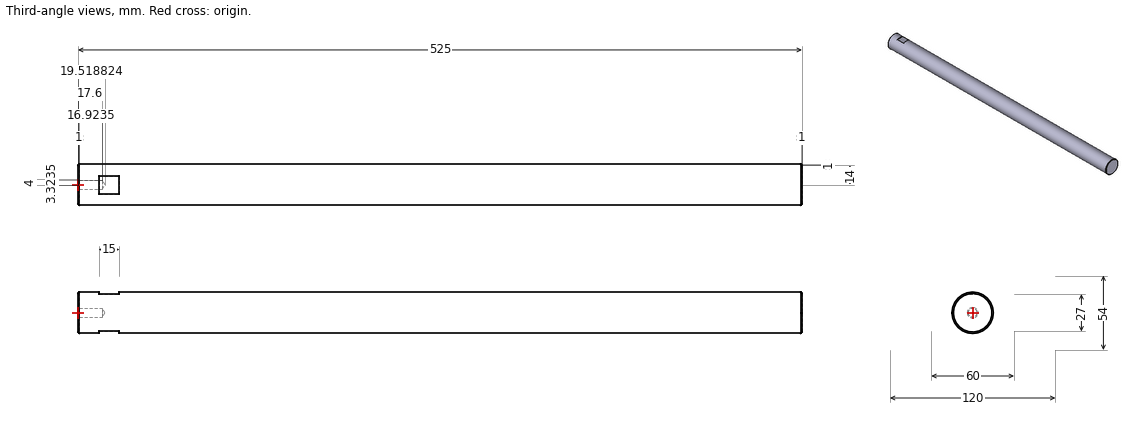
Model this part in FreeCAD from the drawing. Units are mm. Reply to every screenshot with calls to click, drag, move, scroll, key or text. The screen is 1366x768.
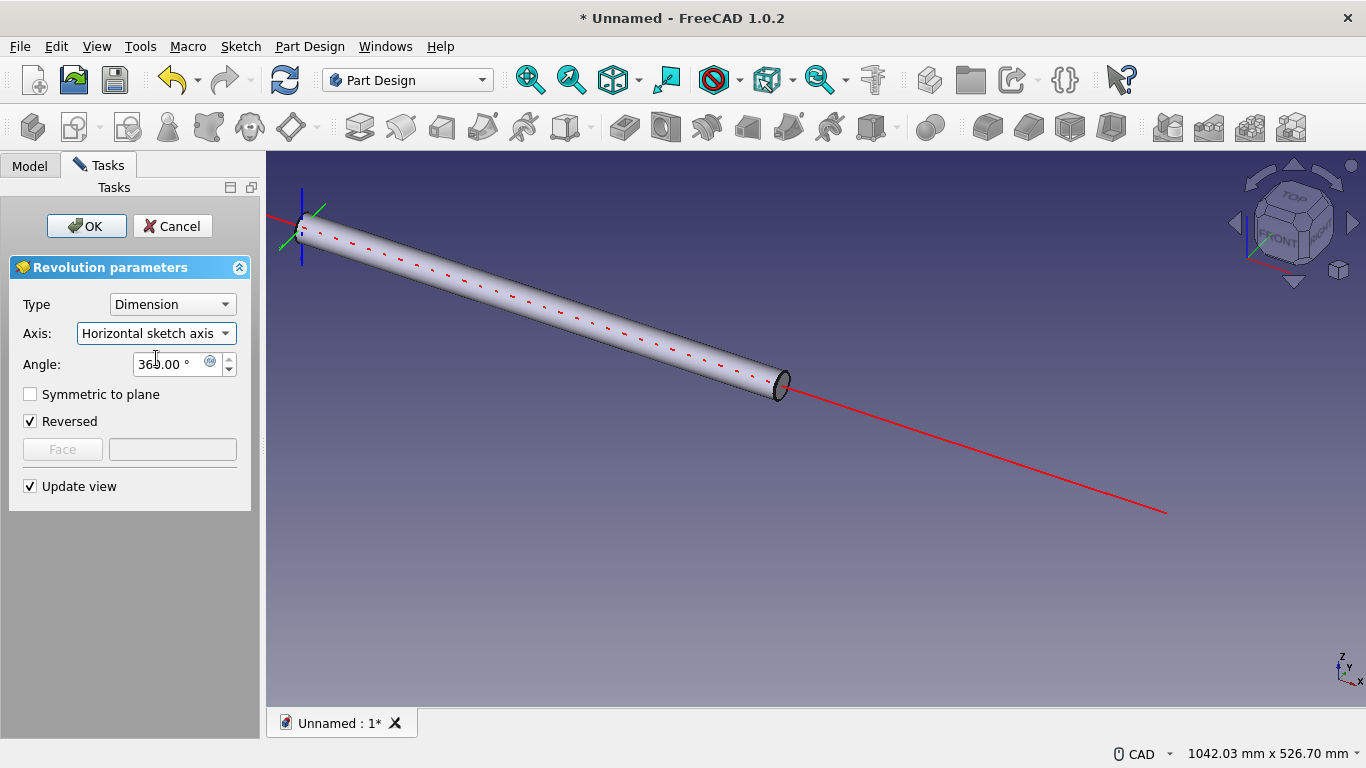
click(87, 226)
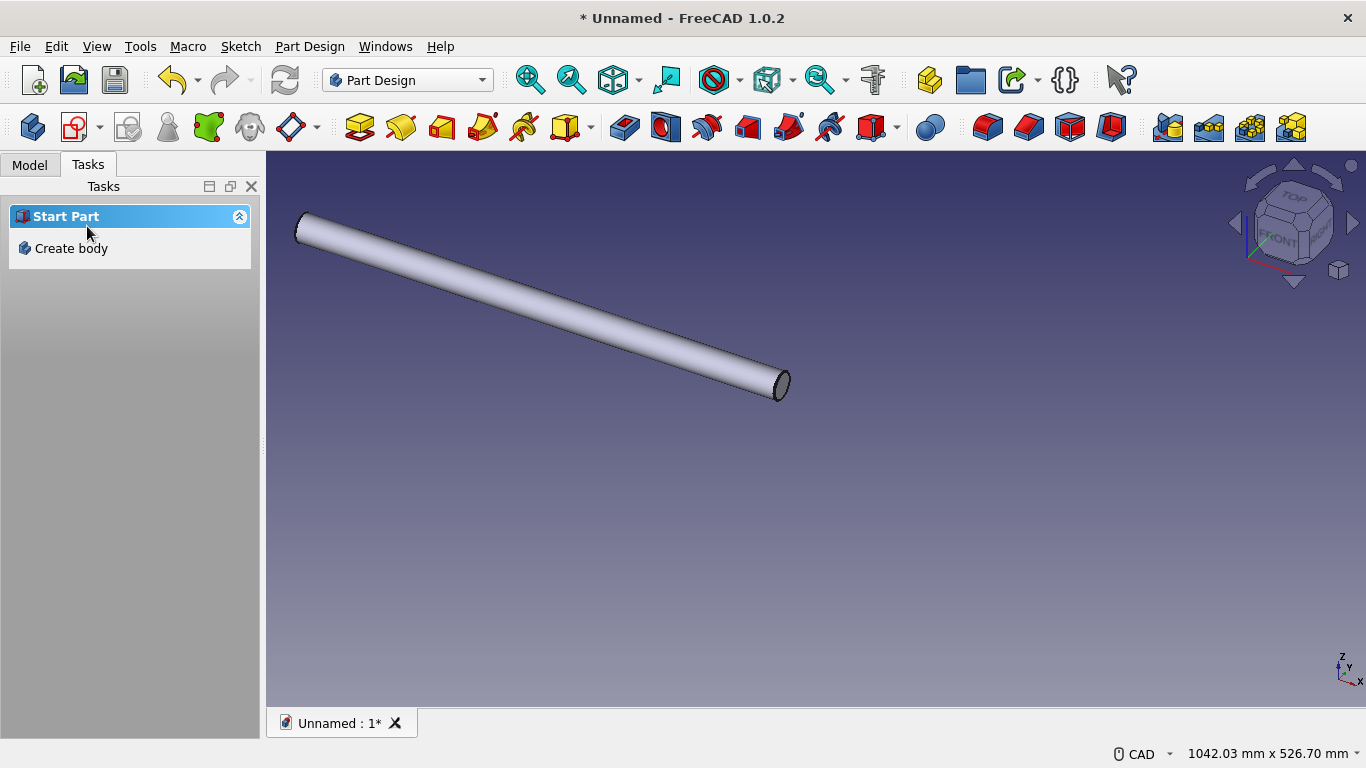
click(30, 164)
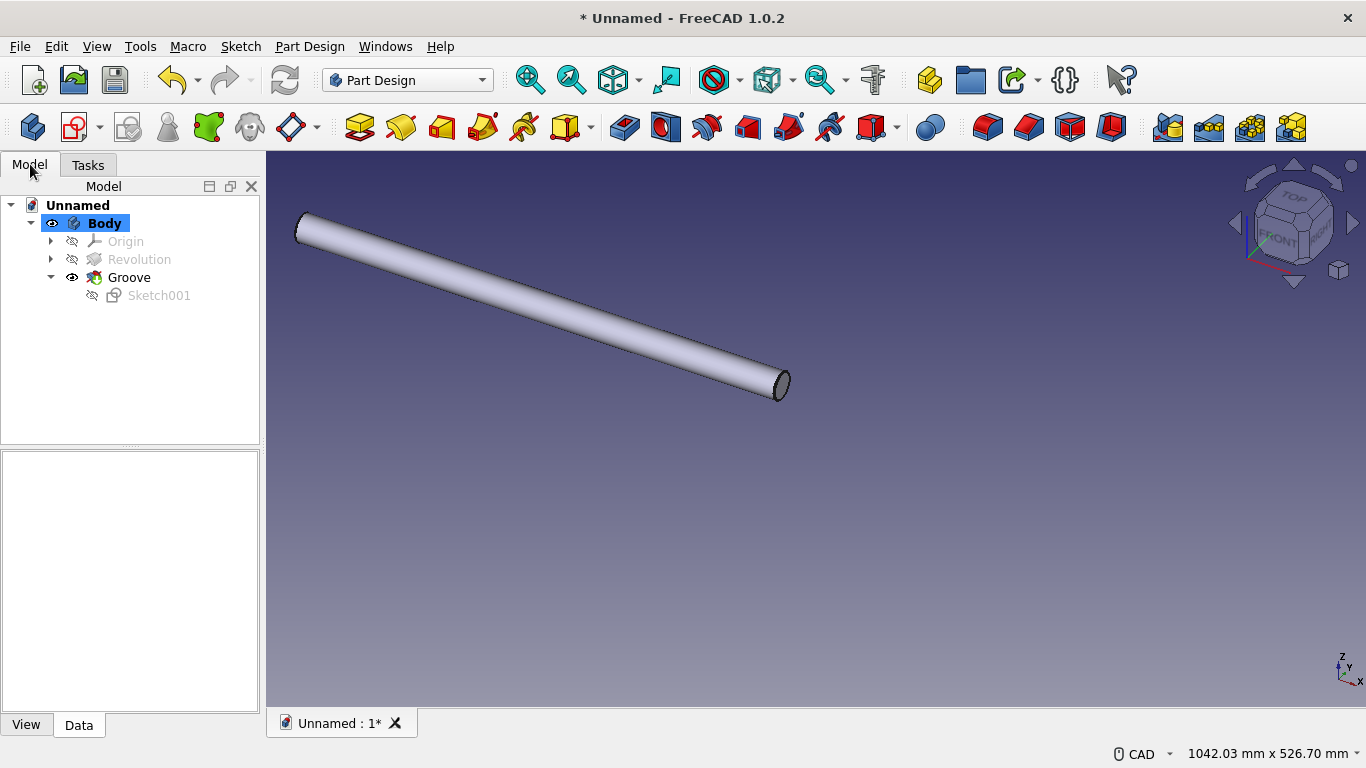
click(51, 241)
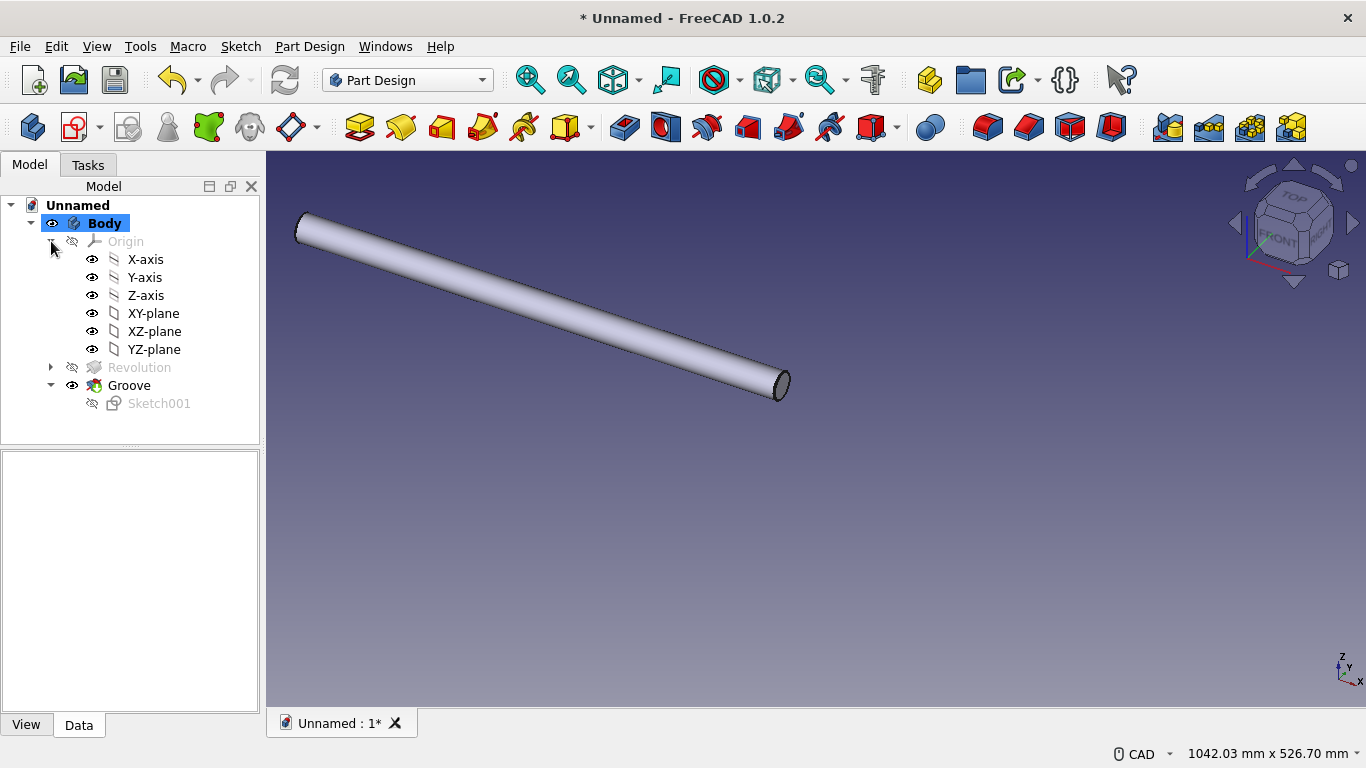
click(137, 349)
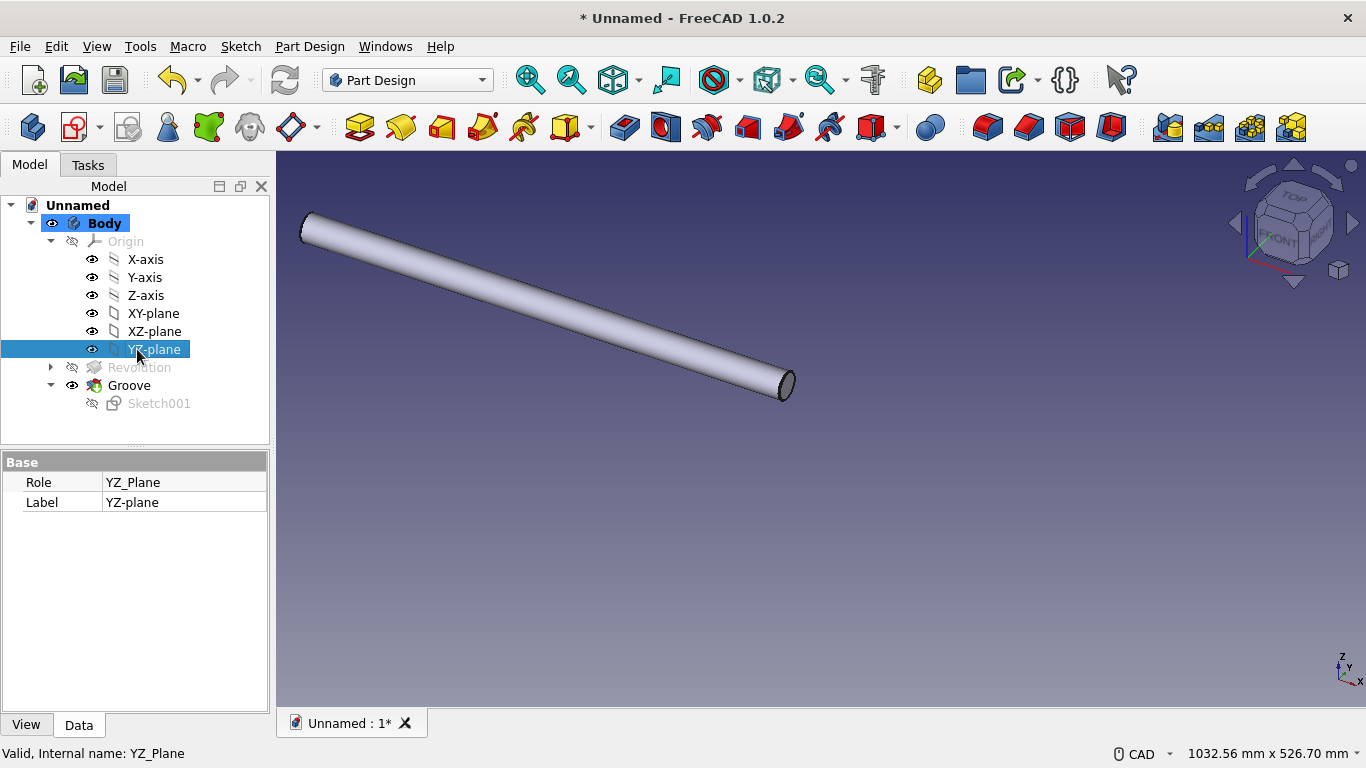
click(290, 128)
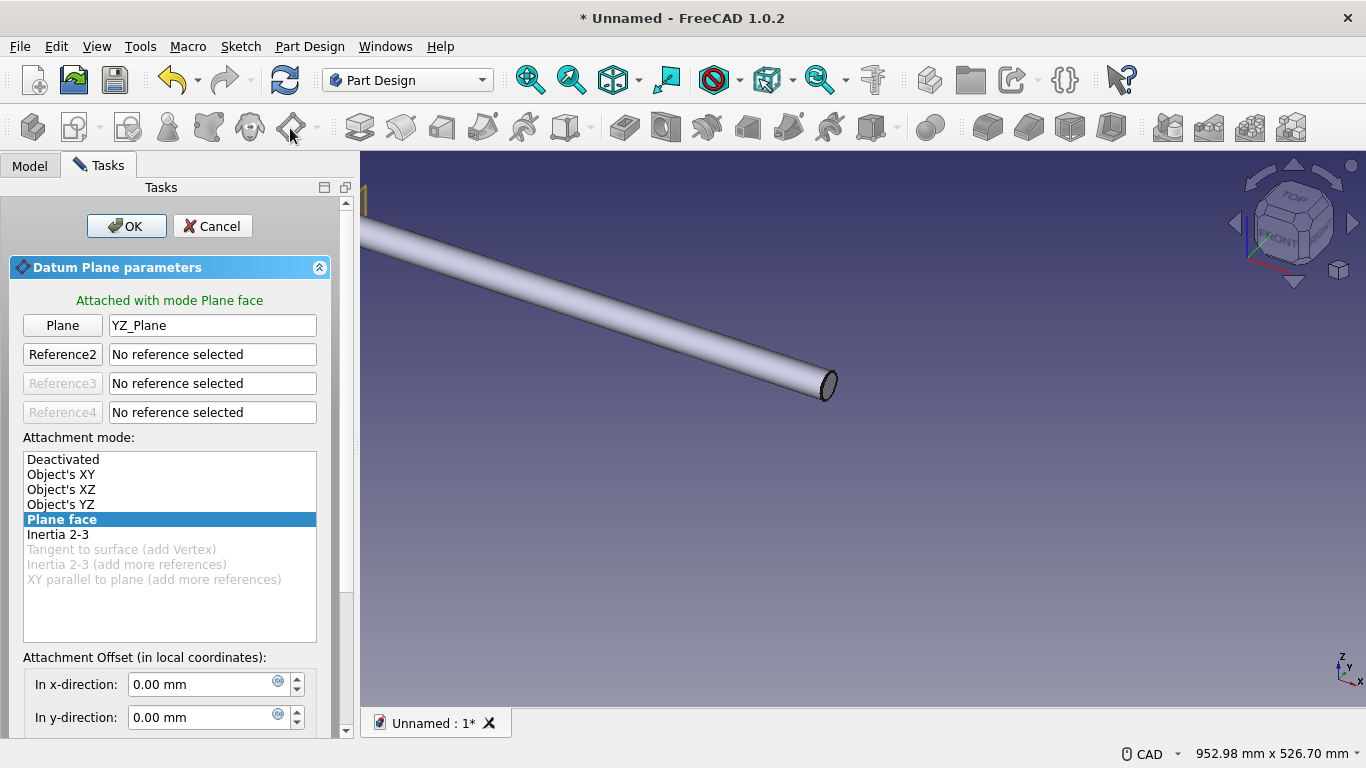
scroll(346, 468, down, 2)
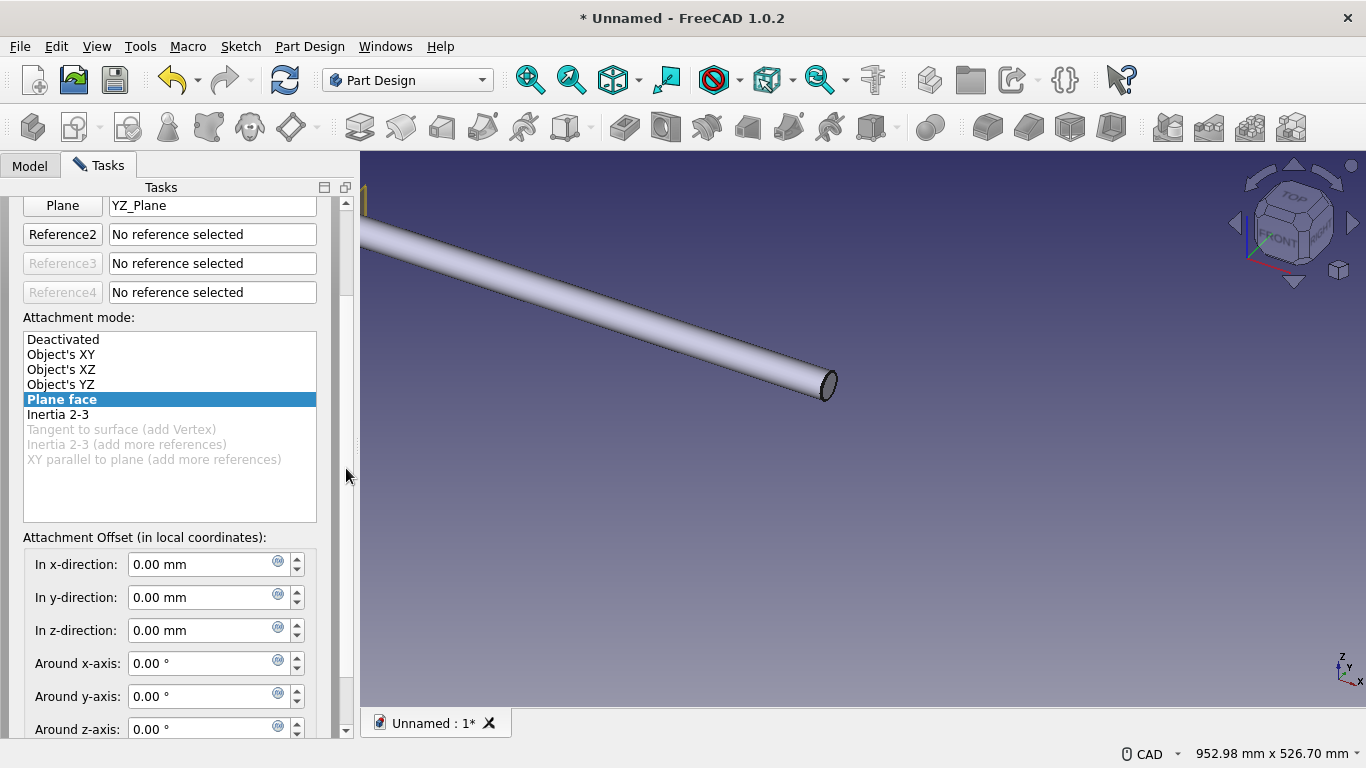
triple_click(210, 630)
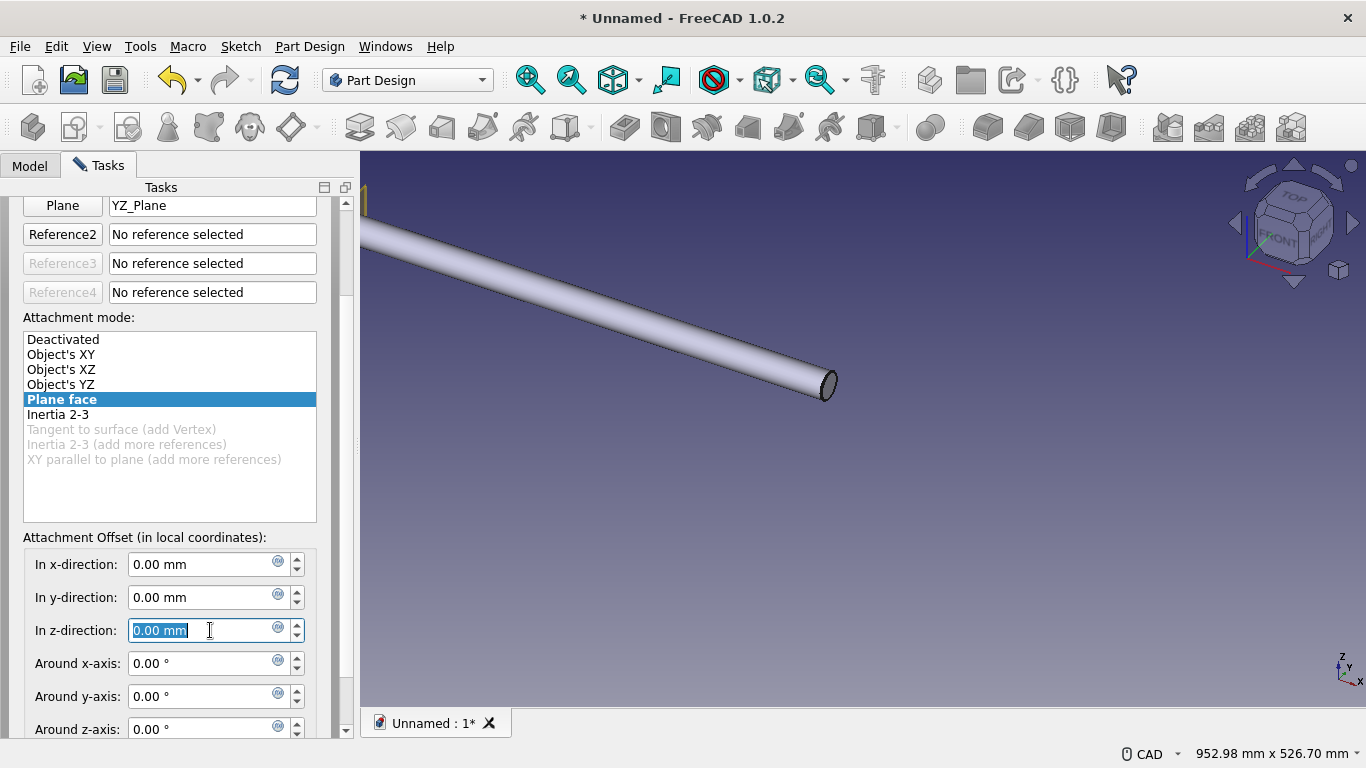
text(15)
key(Tab)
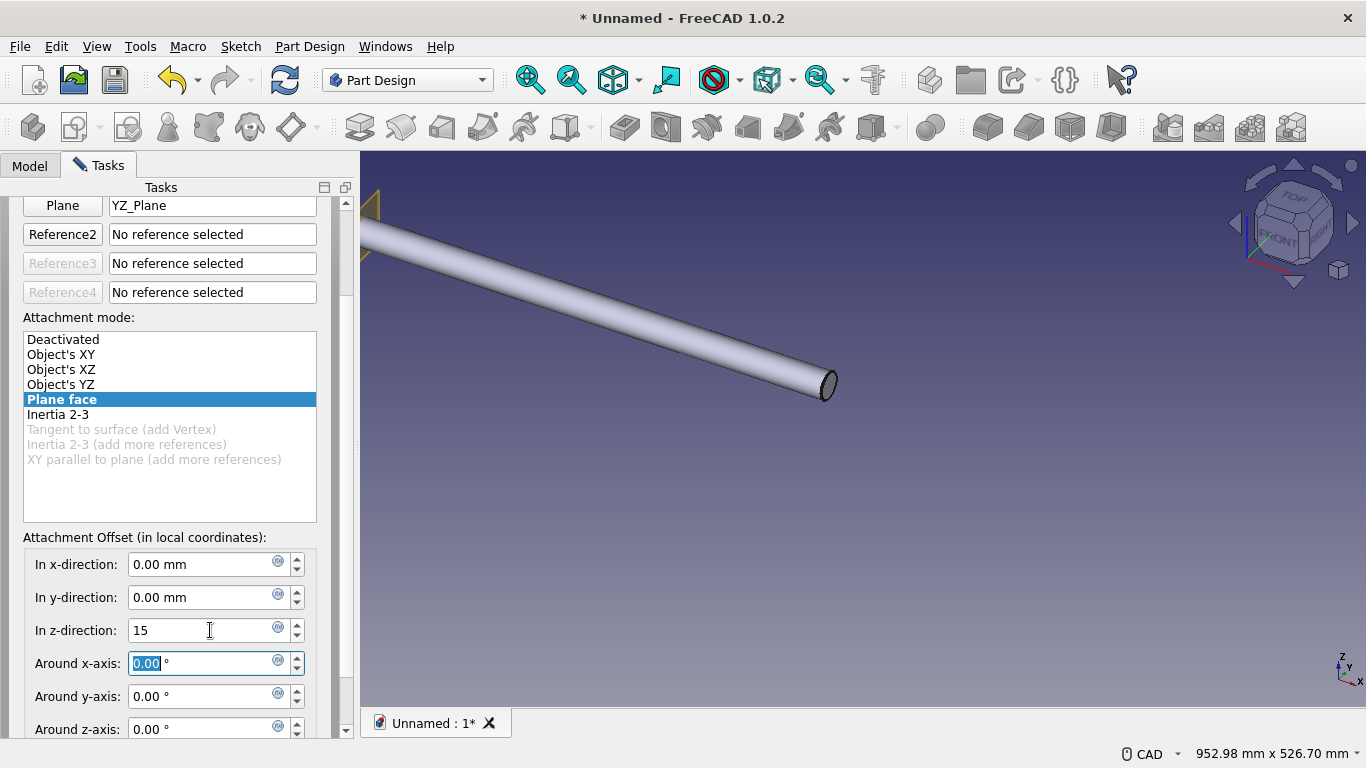
scroll(346, 468, up, 3)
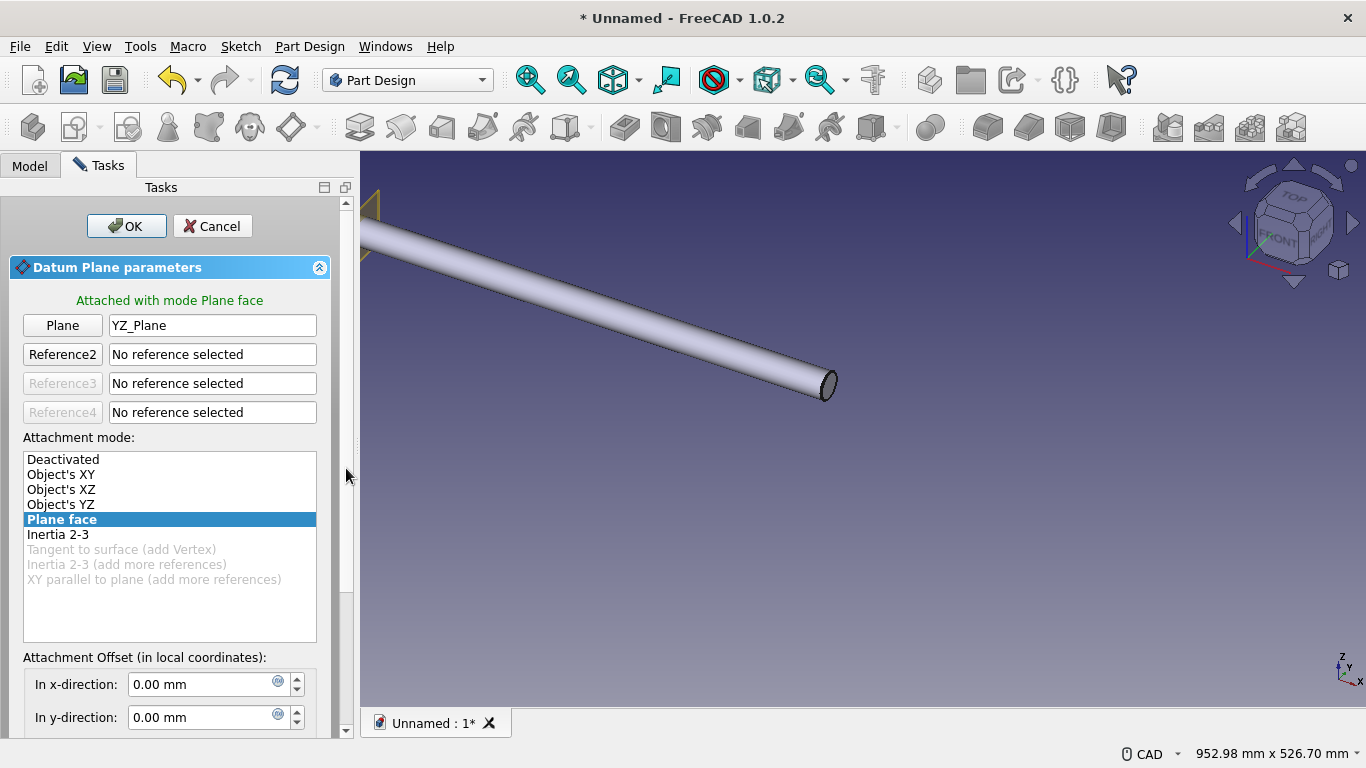
click(127, 226)